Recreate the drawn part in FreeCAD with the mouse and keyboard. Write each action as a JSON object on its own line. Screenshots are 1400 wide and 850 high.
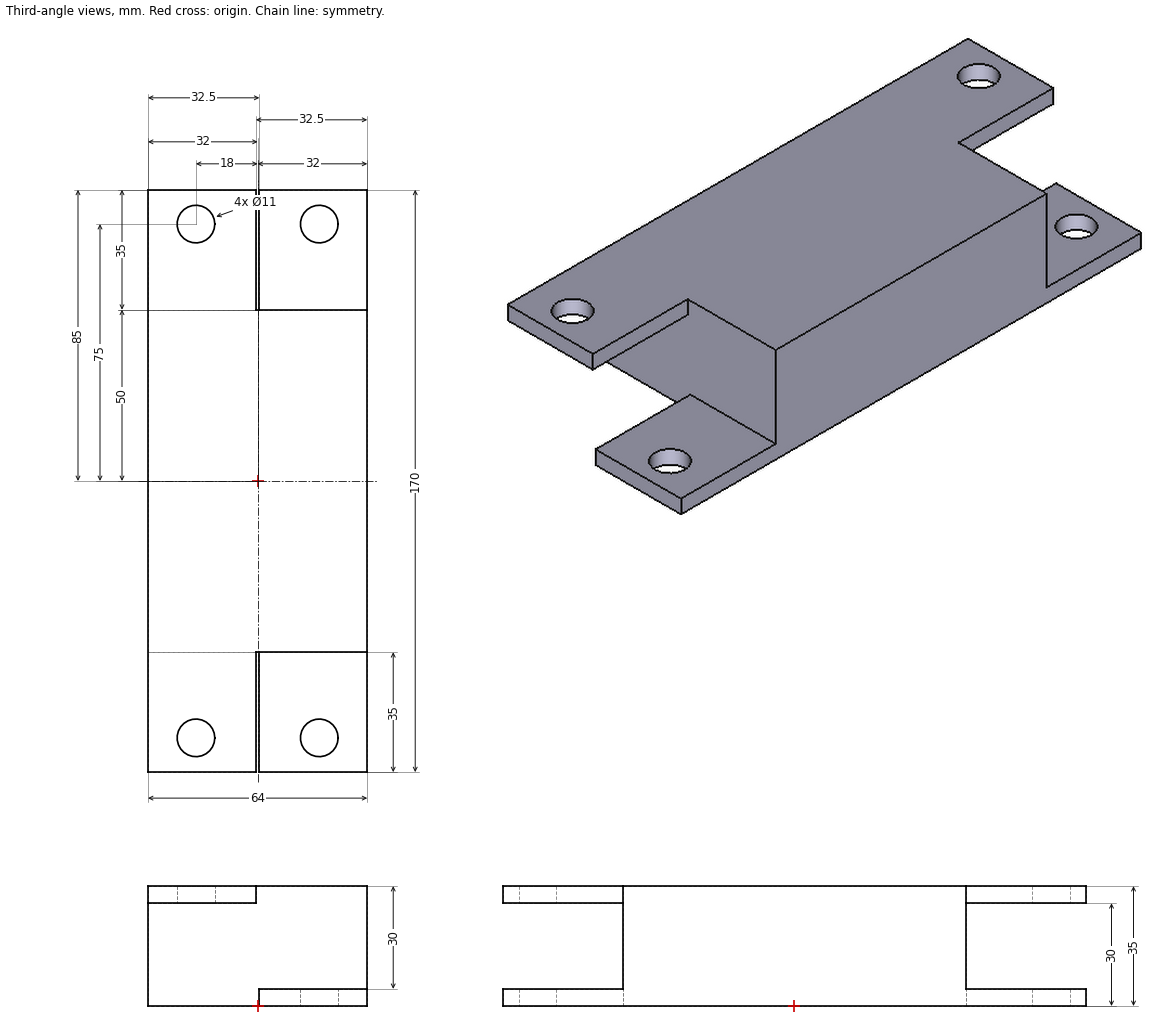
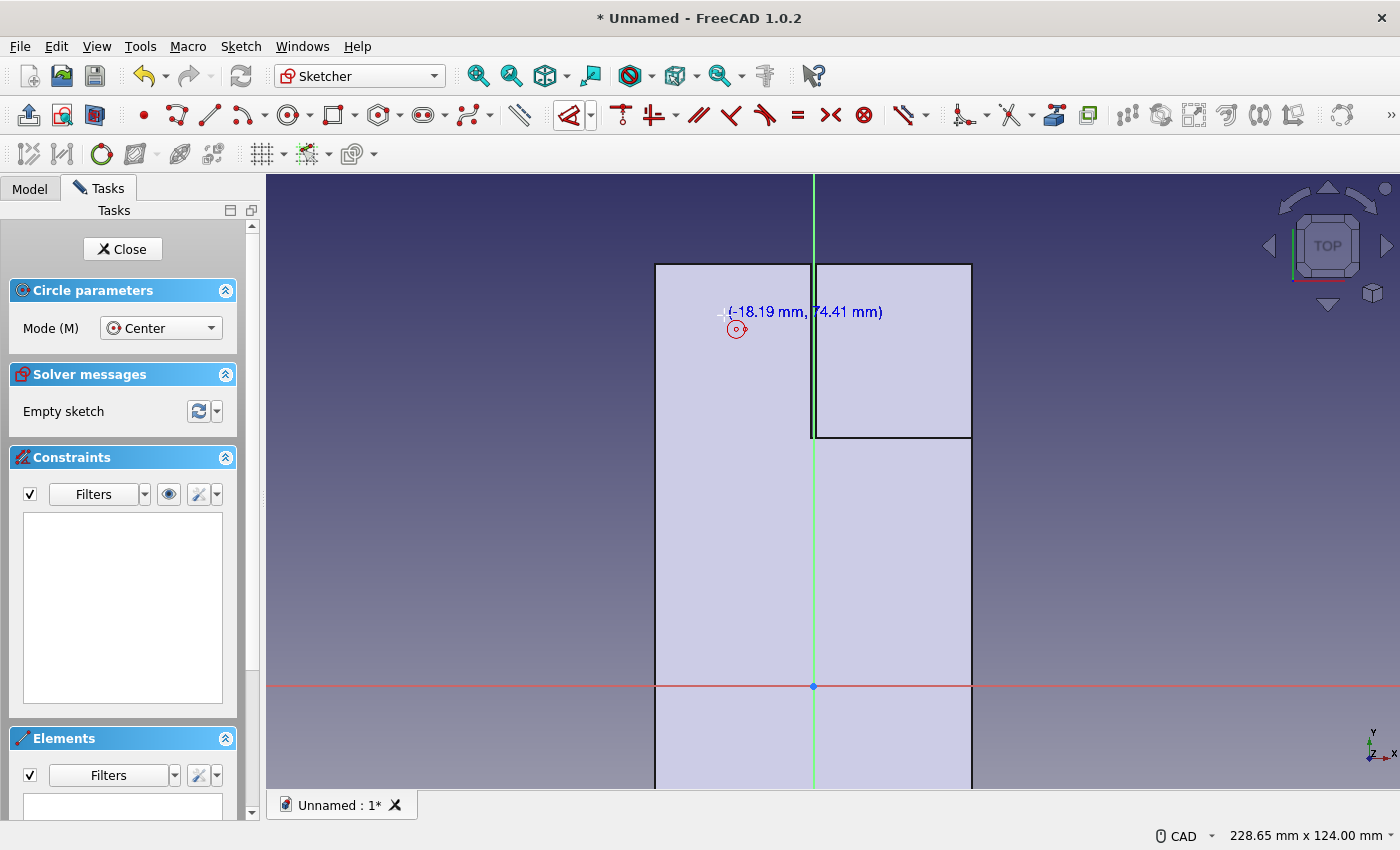
{"action": "left_click", "coordinate": [724, 314]}
{"action": "mouse_move", "coordinate": [744, 295]}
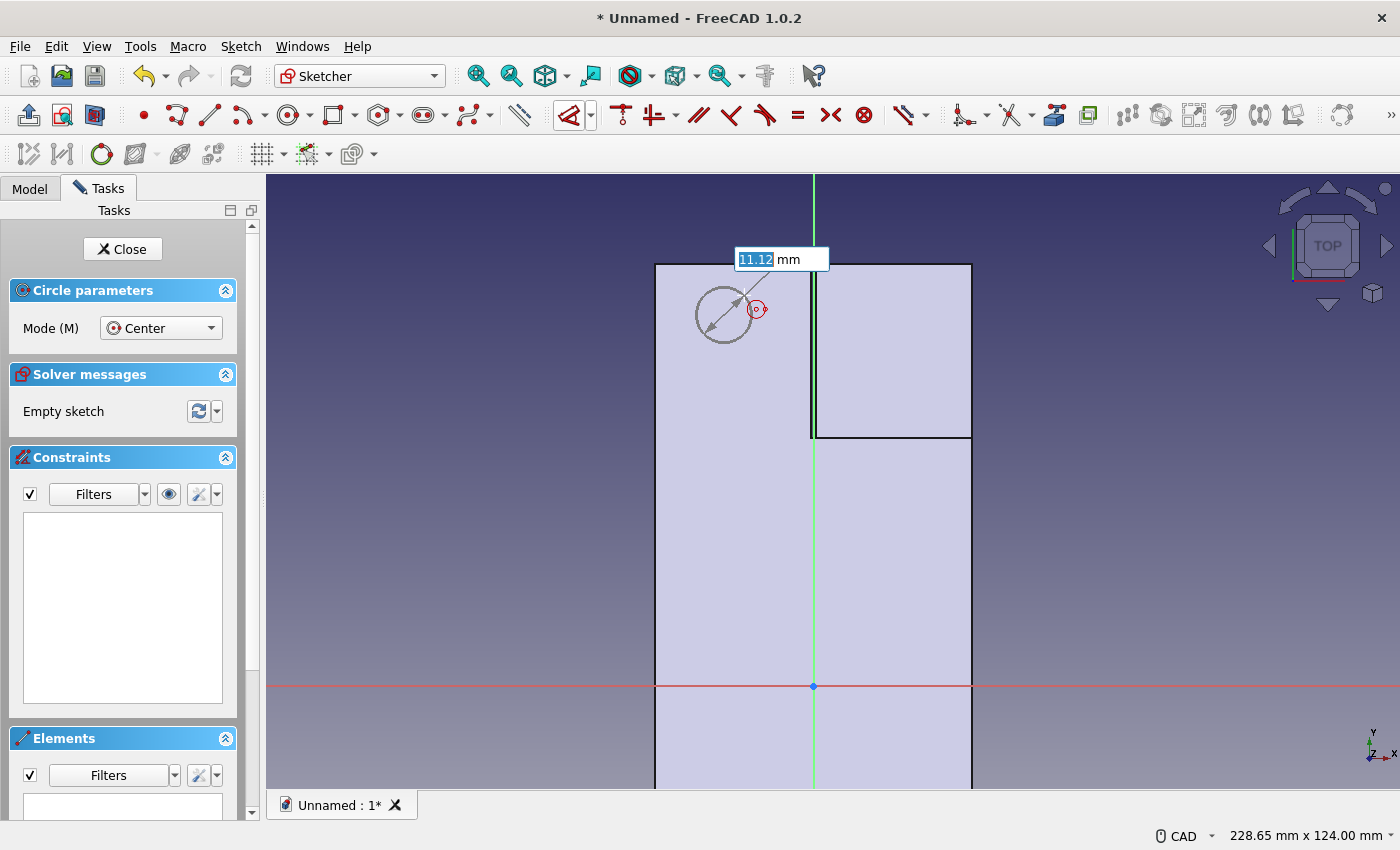
{"action": "type", "text": "11"}
{"action": "key", "text": "Return"}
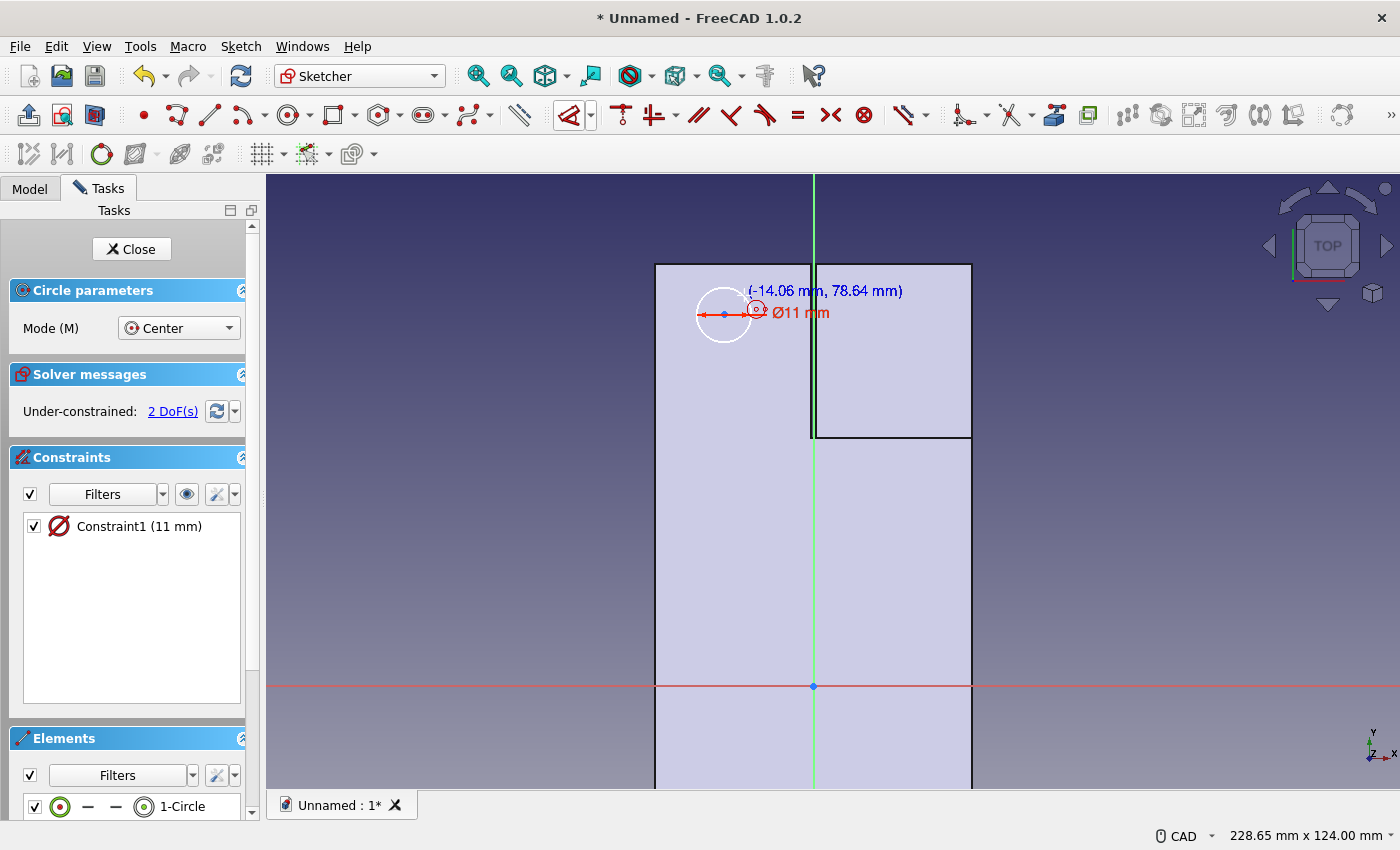
{"action": "left_click", "coordinate": [903, 314]}
{"action": "mouse_move", "coordinate": [922, 295]}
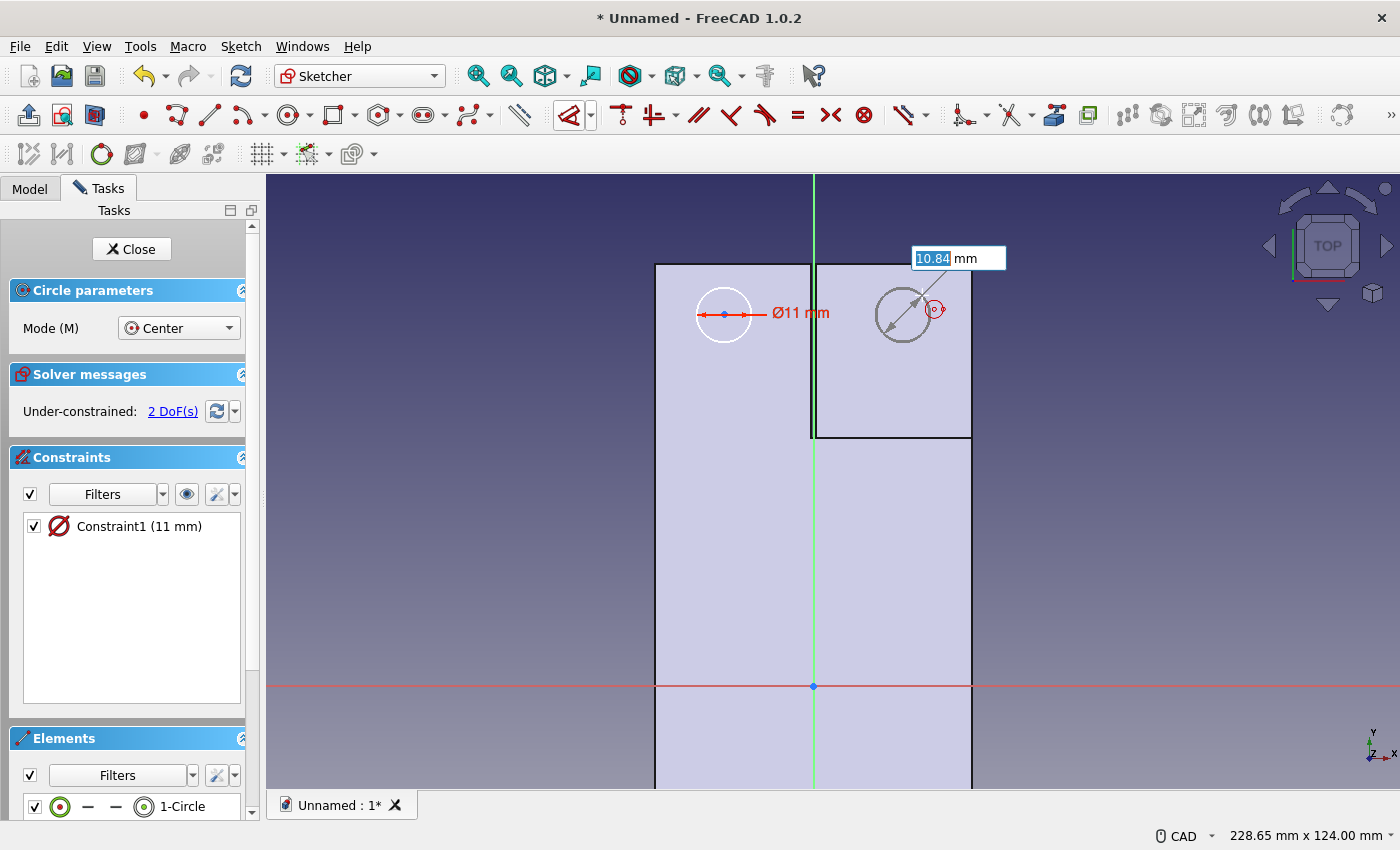
{"action": "type", "text": "11"}
{"action": "key", "text": "Return"}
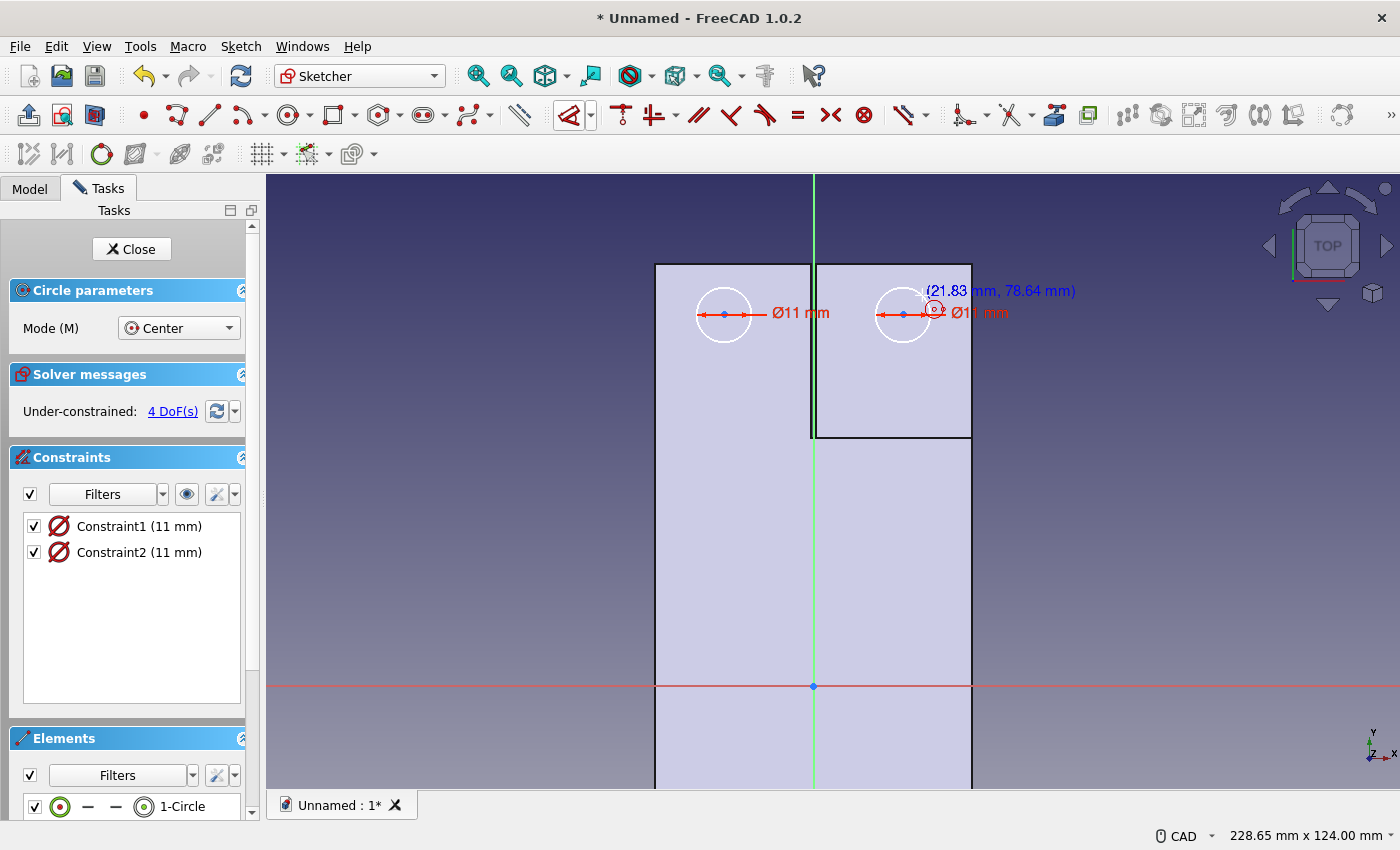
{"action": "scroll", "coordinate": [724, 315], "scroll_direction": "down", "scroll_amount": 4}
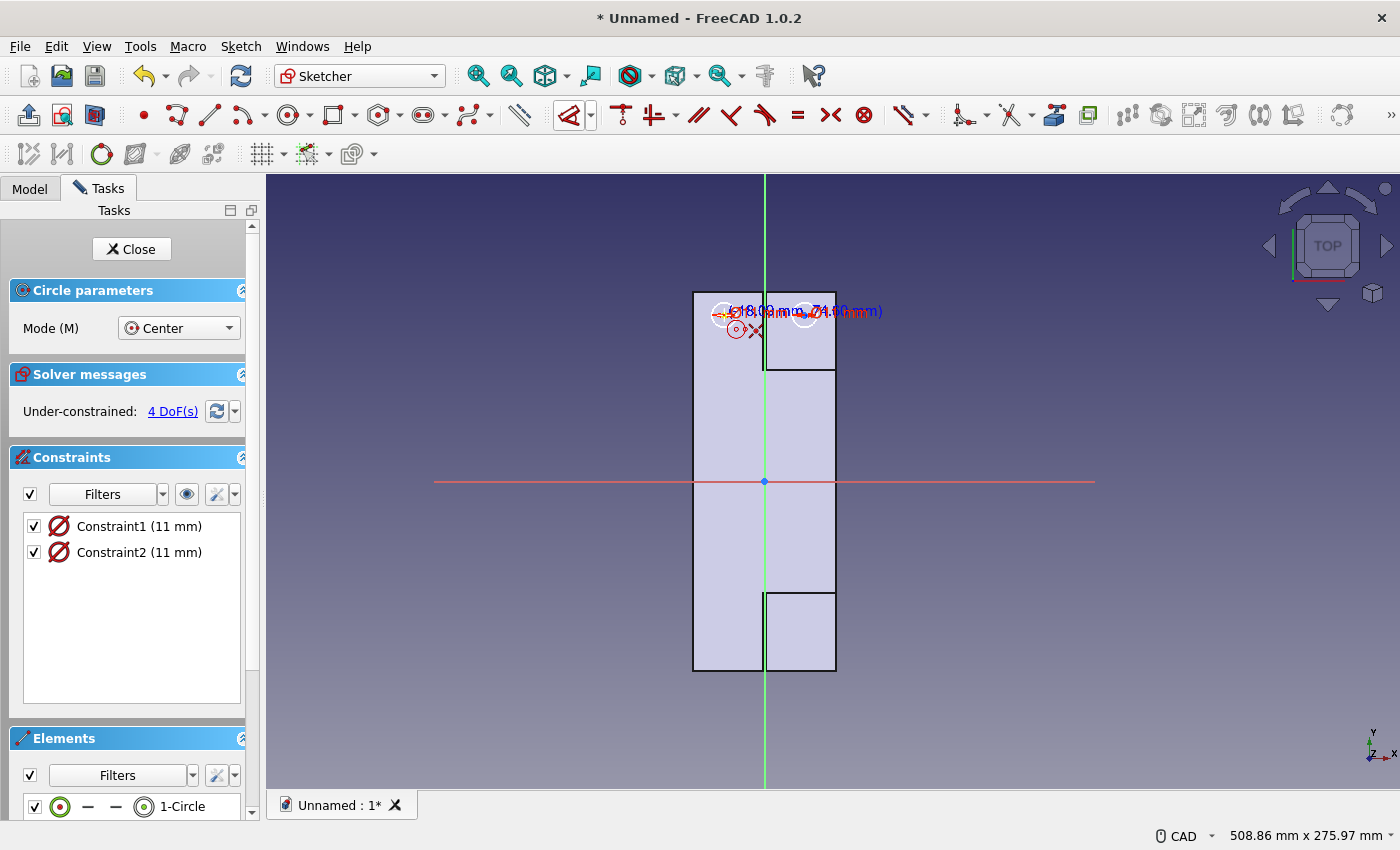
{"action": "scroll", "coordinate": [805, 649], "scroll_direction": "up", "scroll_amount": 4}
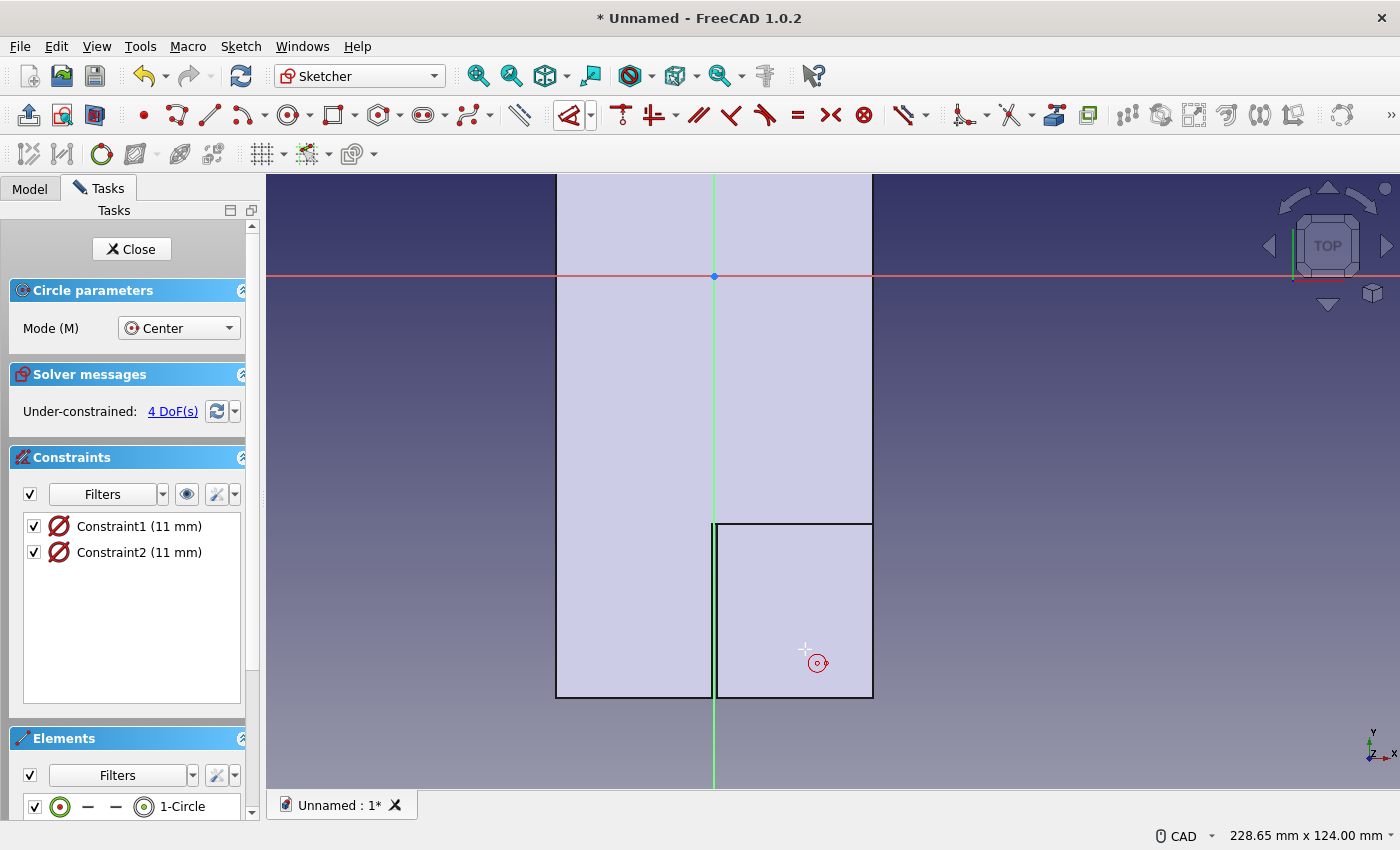
{"action": "left_click", "coordinate": [804, 648]}
{"action": "mouse_move", "coordinate": [823, 629]}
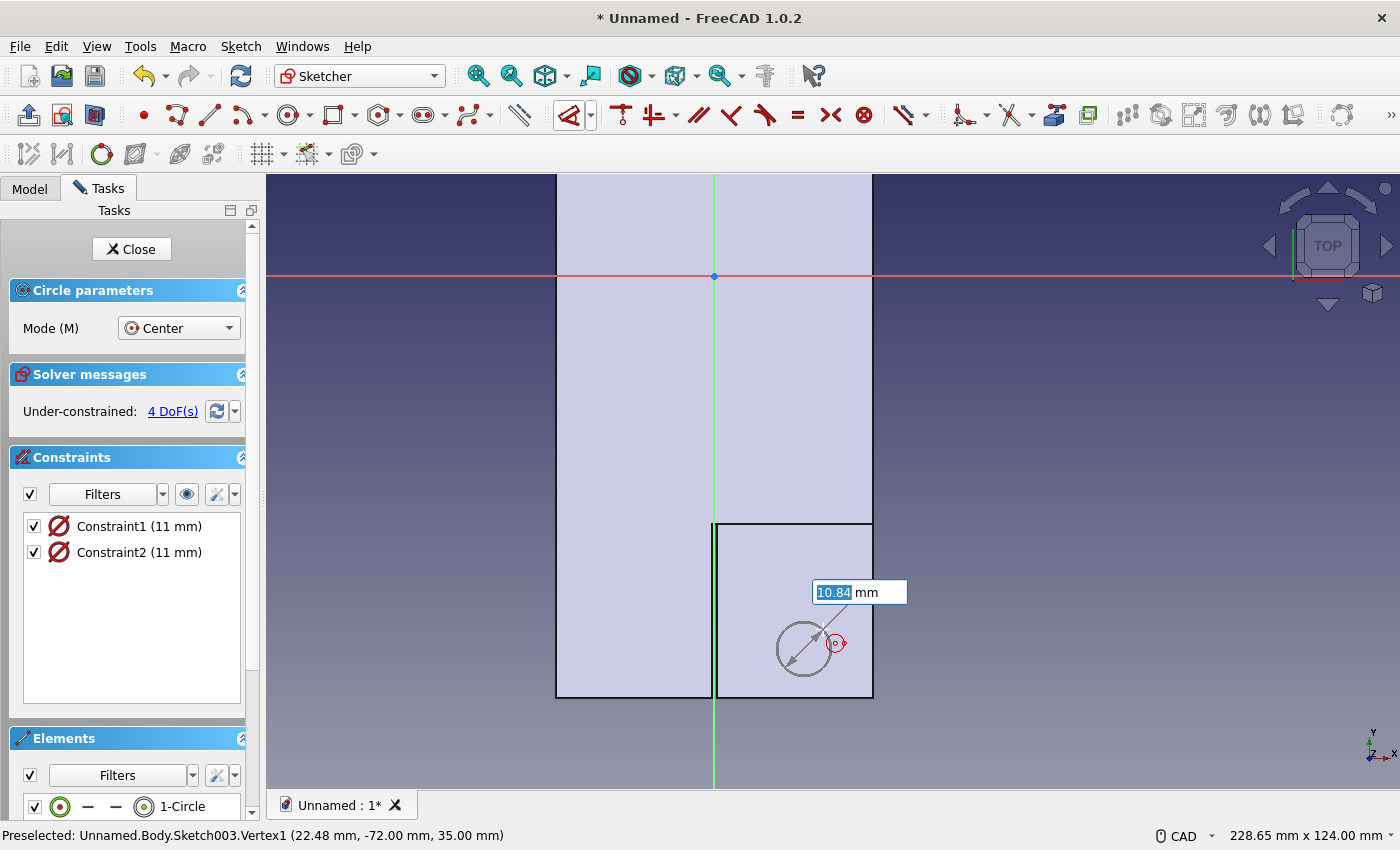
{"action": "type", "text": "11"}
{"action": "key", "text": "Return"}